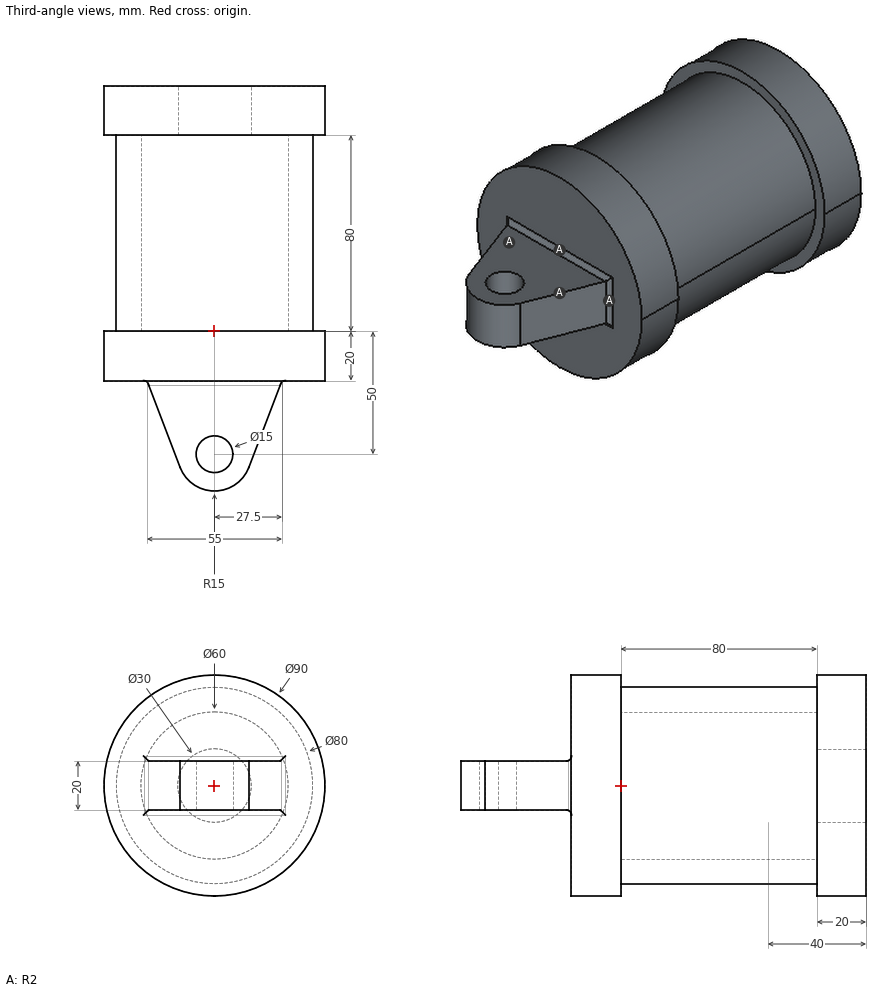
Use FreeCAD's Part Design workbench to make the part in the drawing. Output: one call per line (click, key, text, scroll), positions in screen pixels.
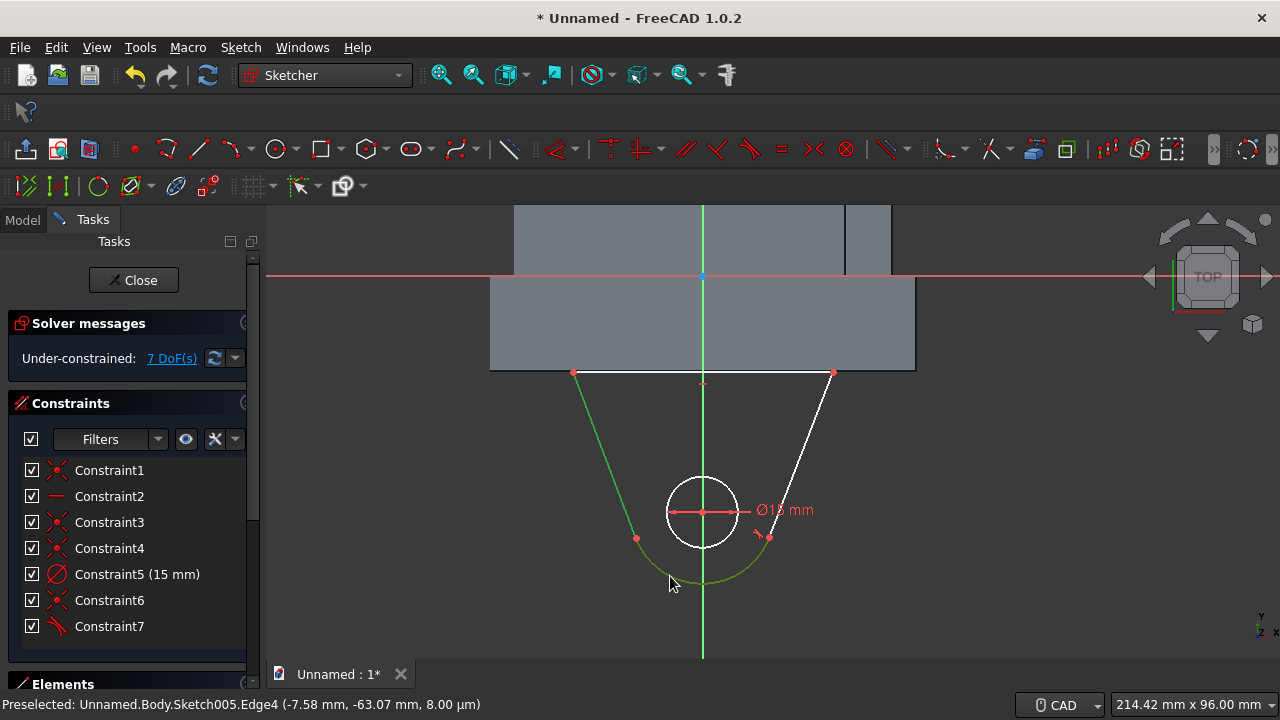
key(t)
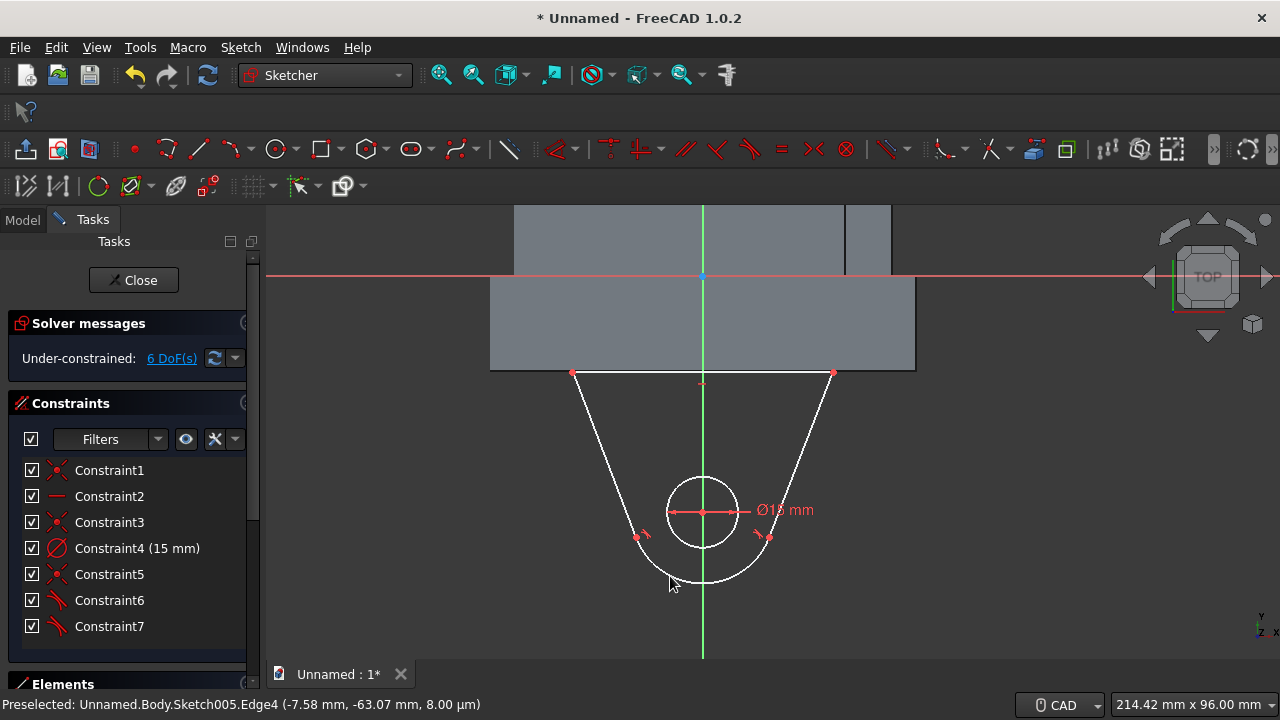
click(703, 512)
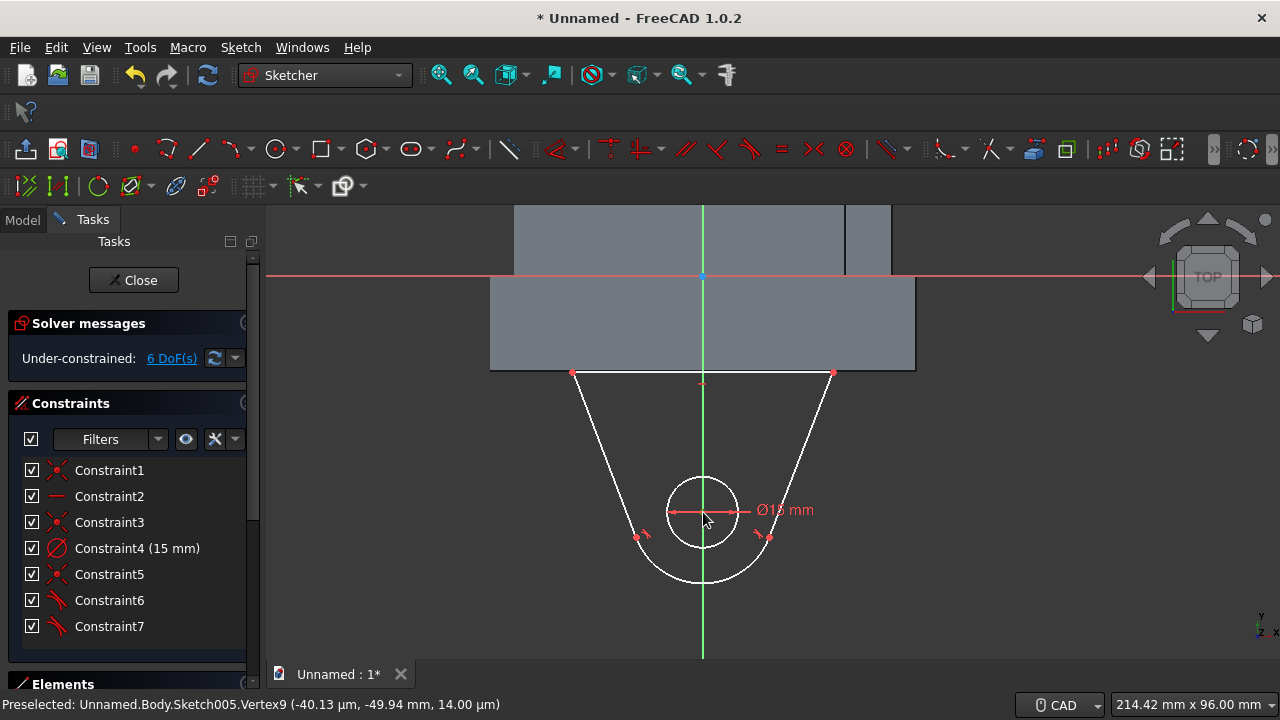
click(703, 517)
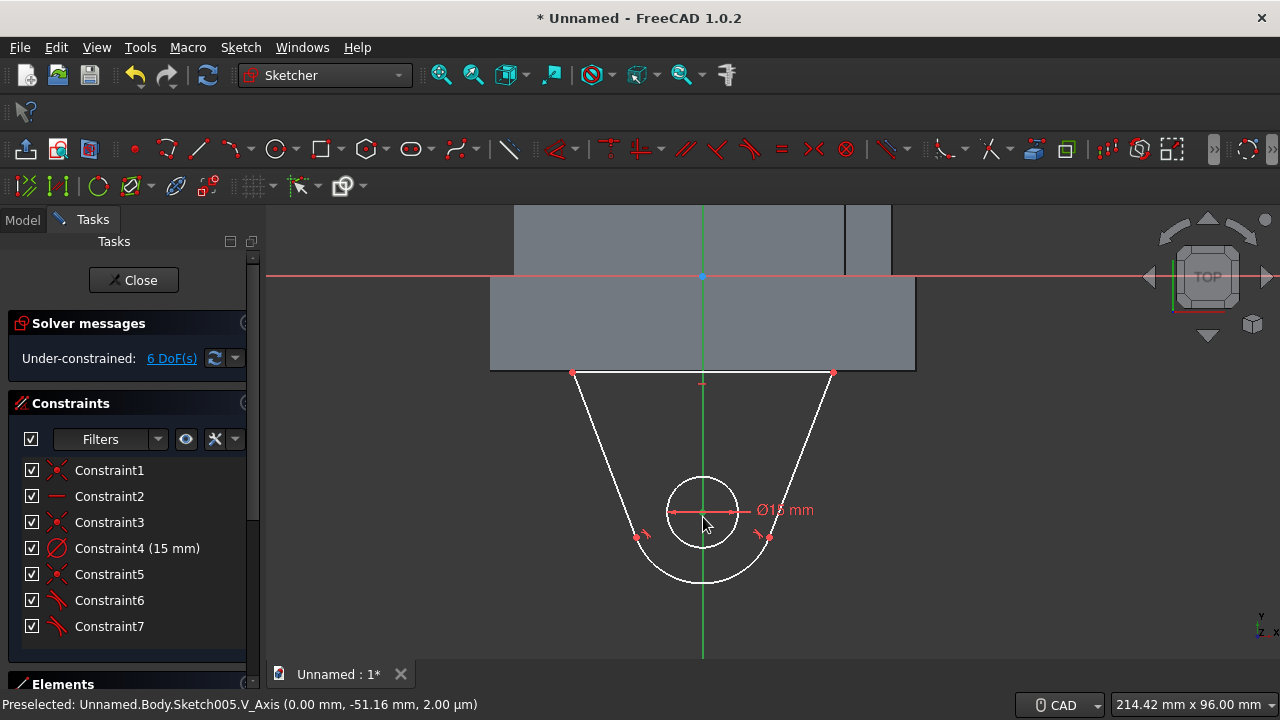
key(c)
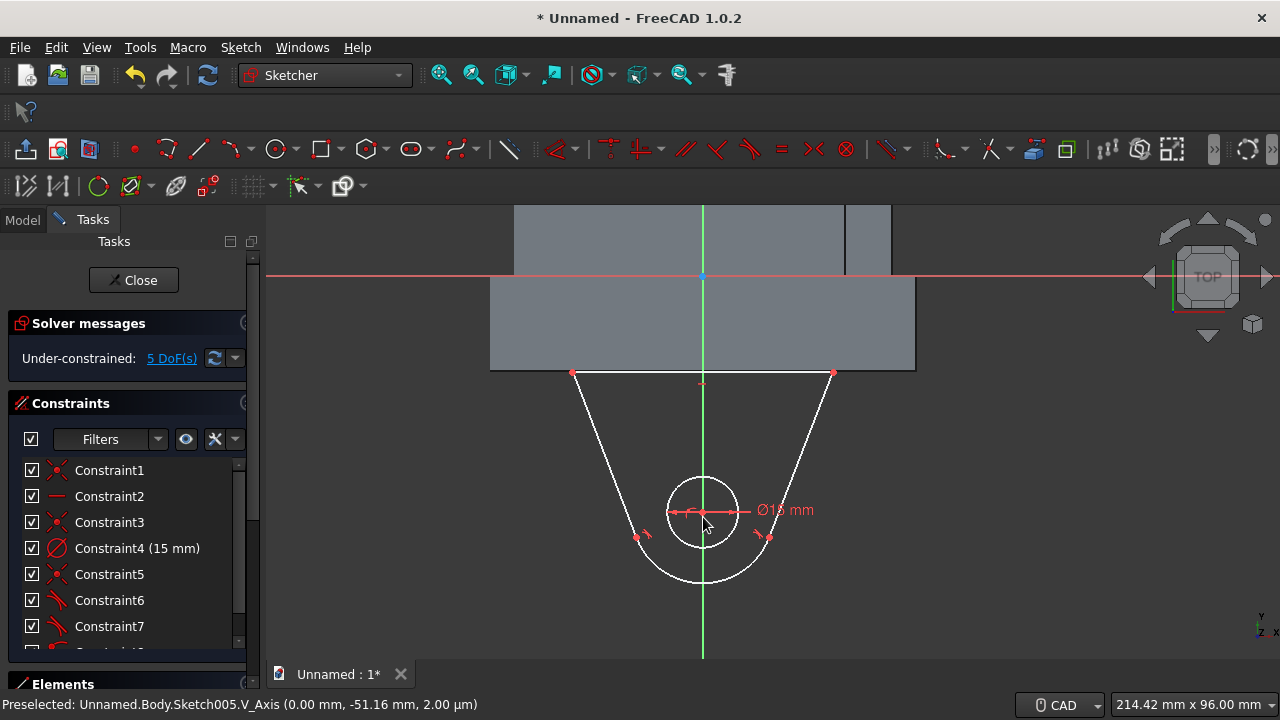
key(d)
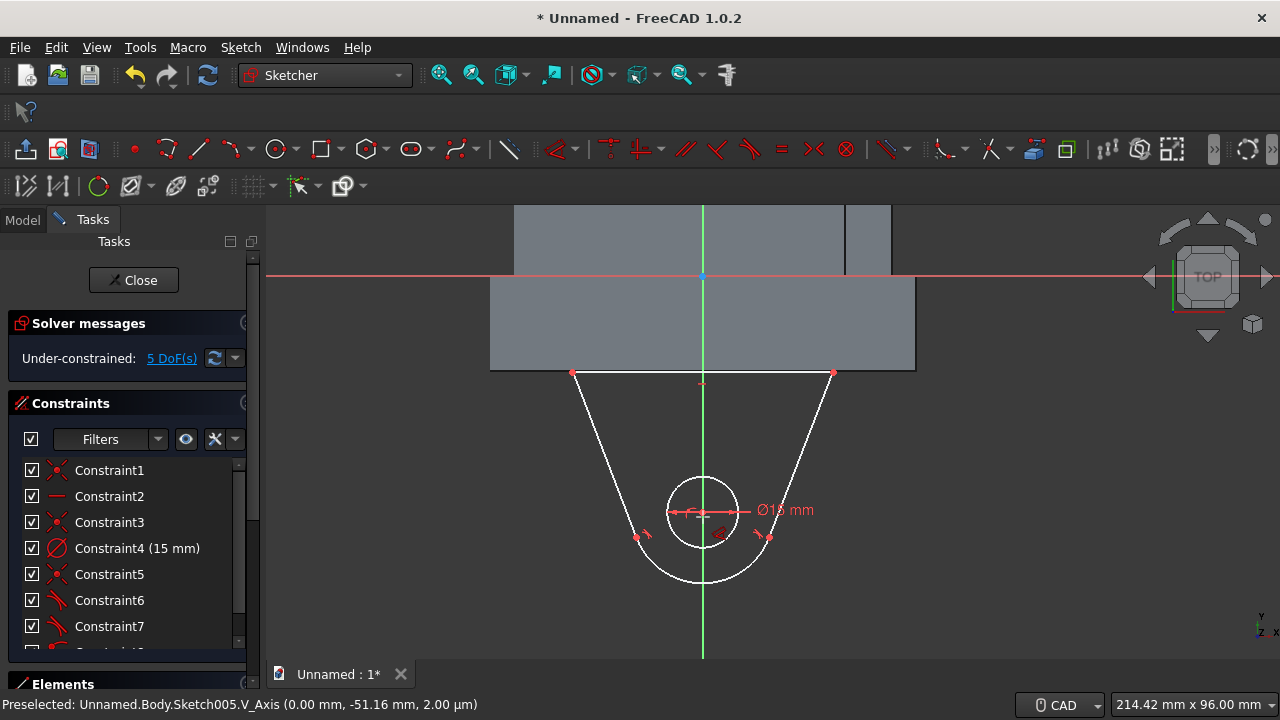
click(670, 575)
click(655, 603)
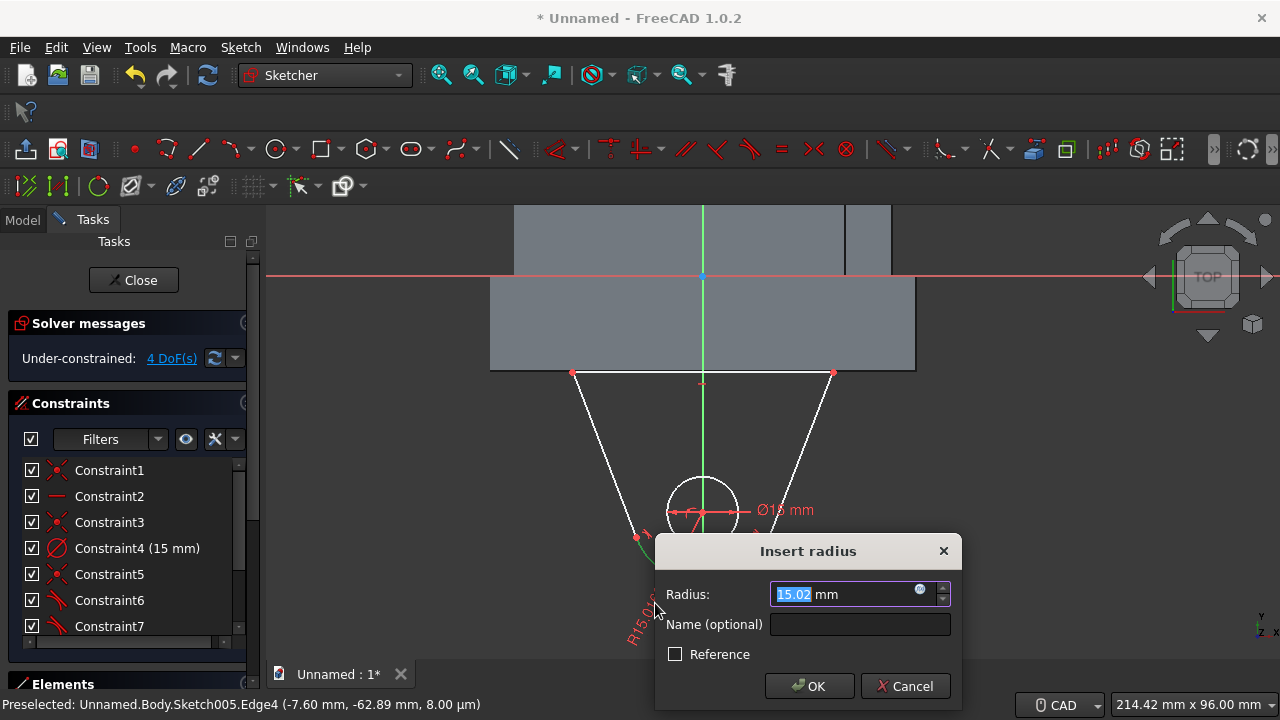
text(15)
key(Return)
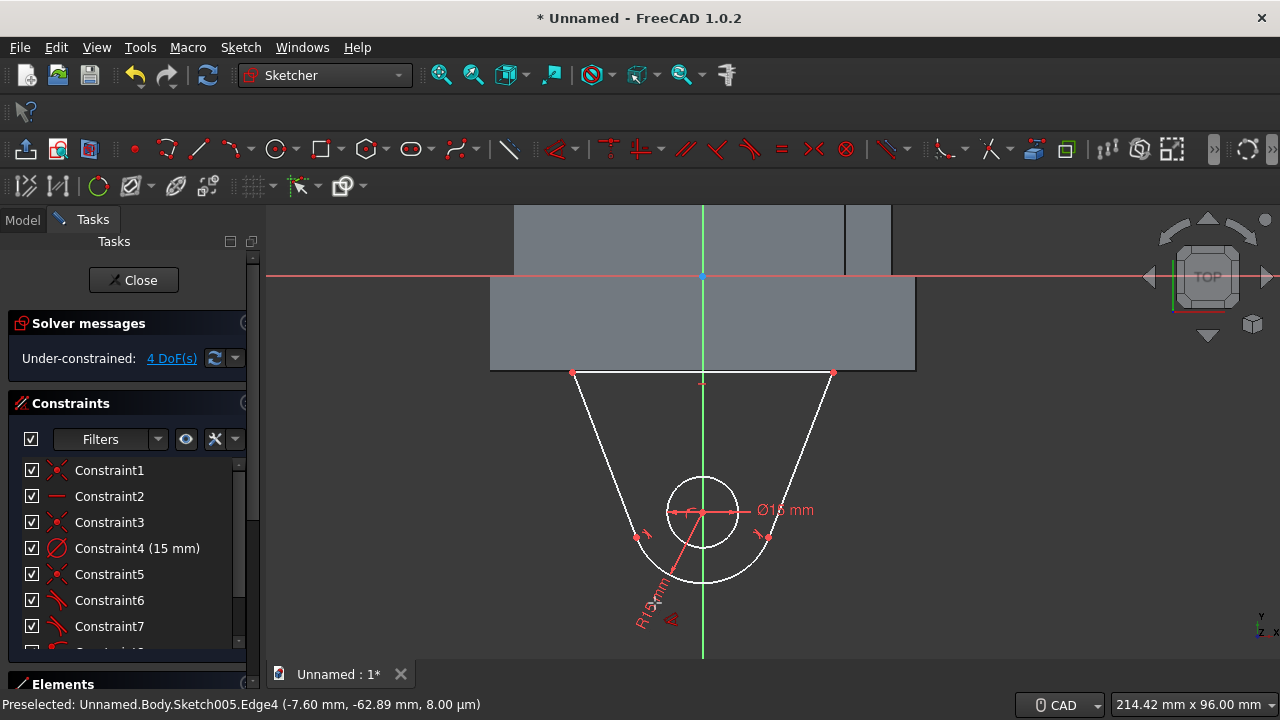
click(755, 372)
click(643, 338)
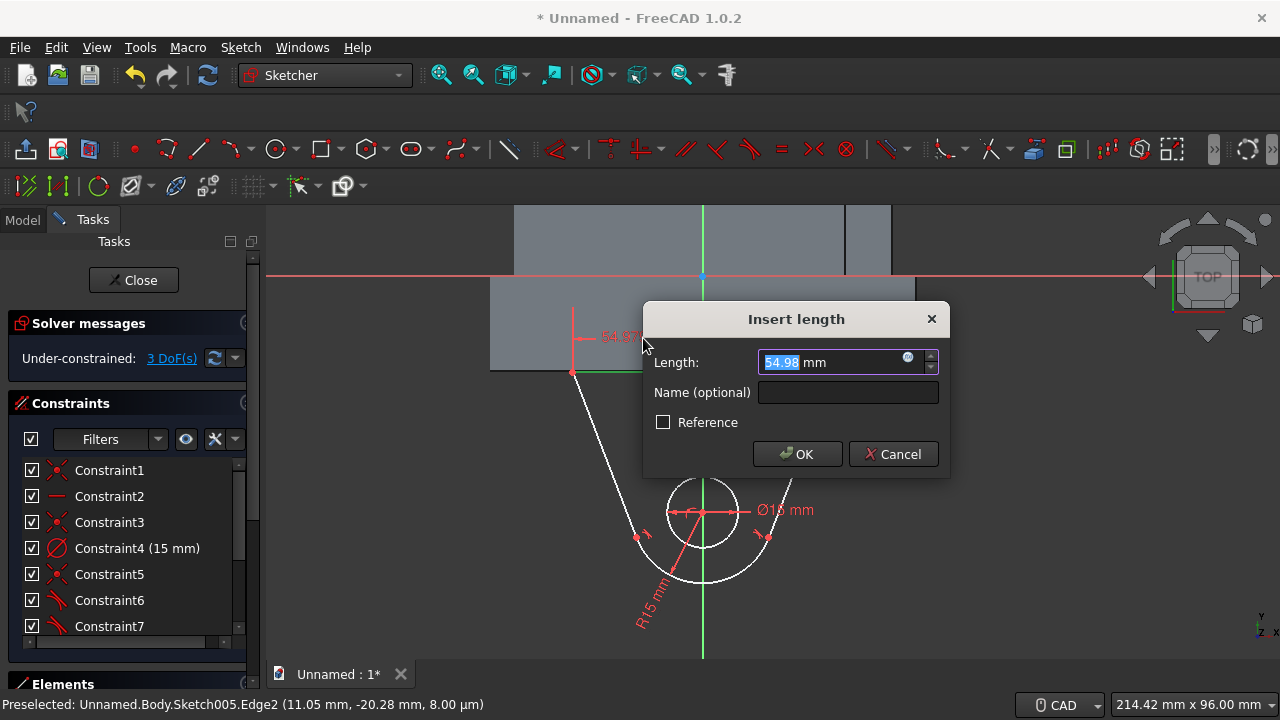
text(55)
key(Return)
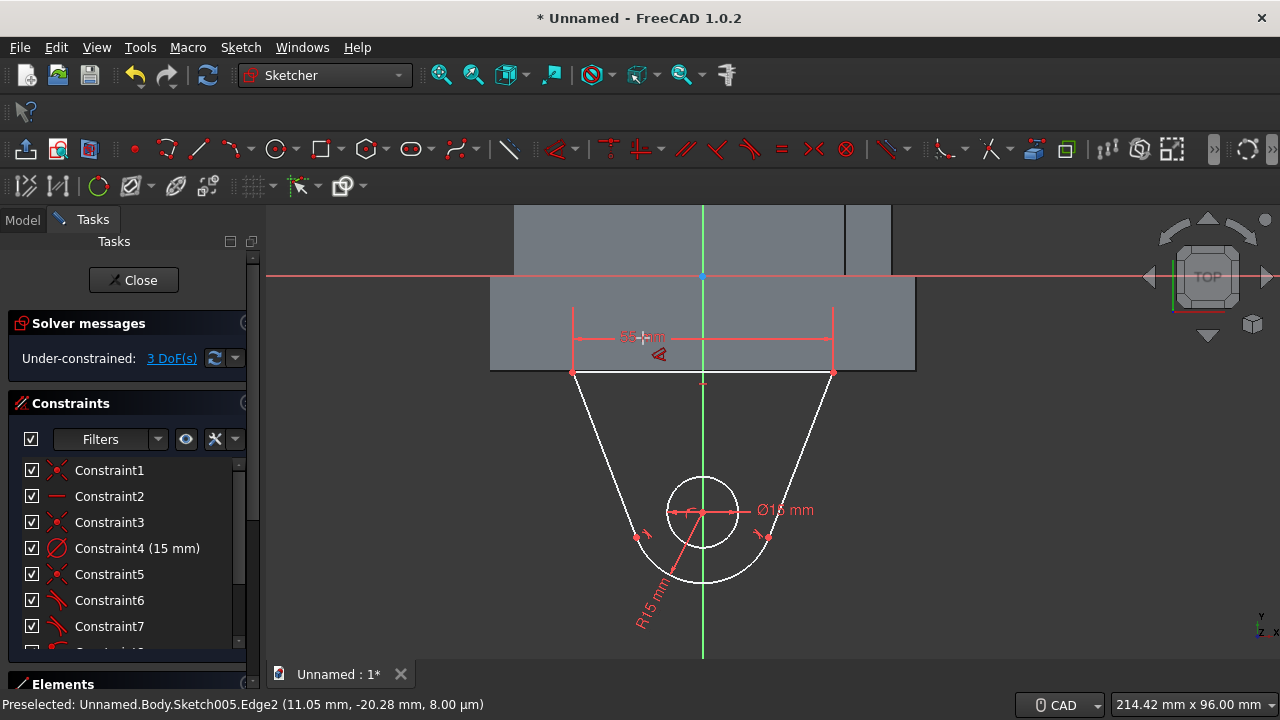
click(703, 512)
click(737, 394)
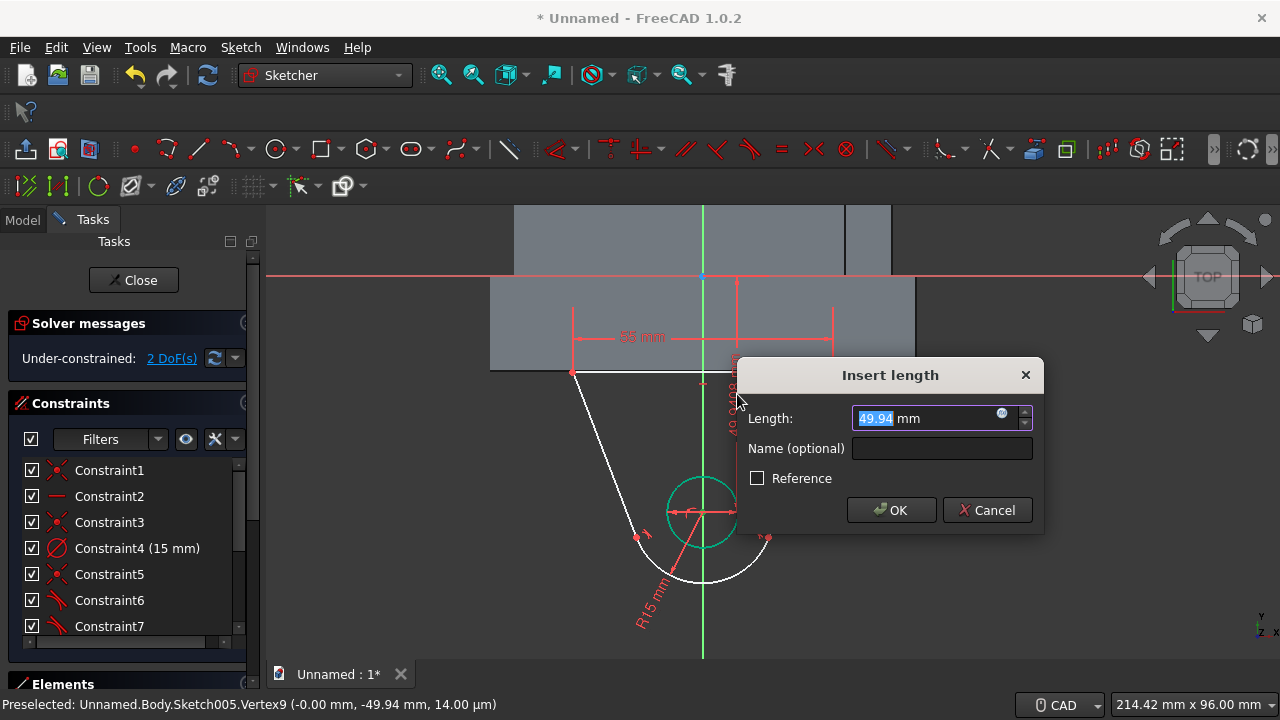
text(50)
key(Return)